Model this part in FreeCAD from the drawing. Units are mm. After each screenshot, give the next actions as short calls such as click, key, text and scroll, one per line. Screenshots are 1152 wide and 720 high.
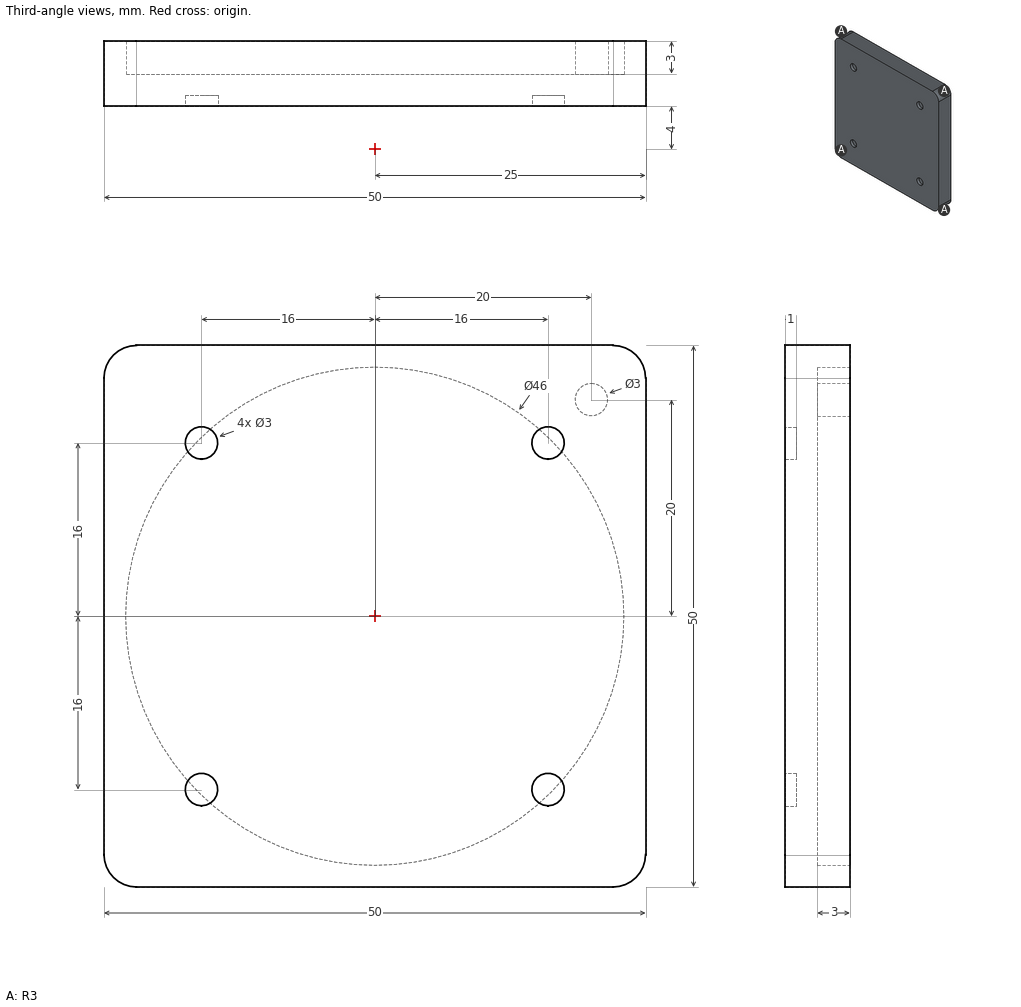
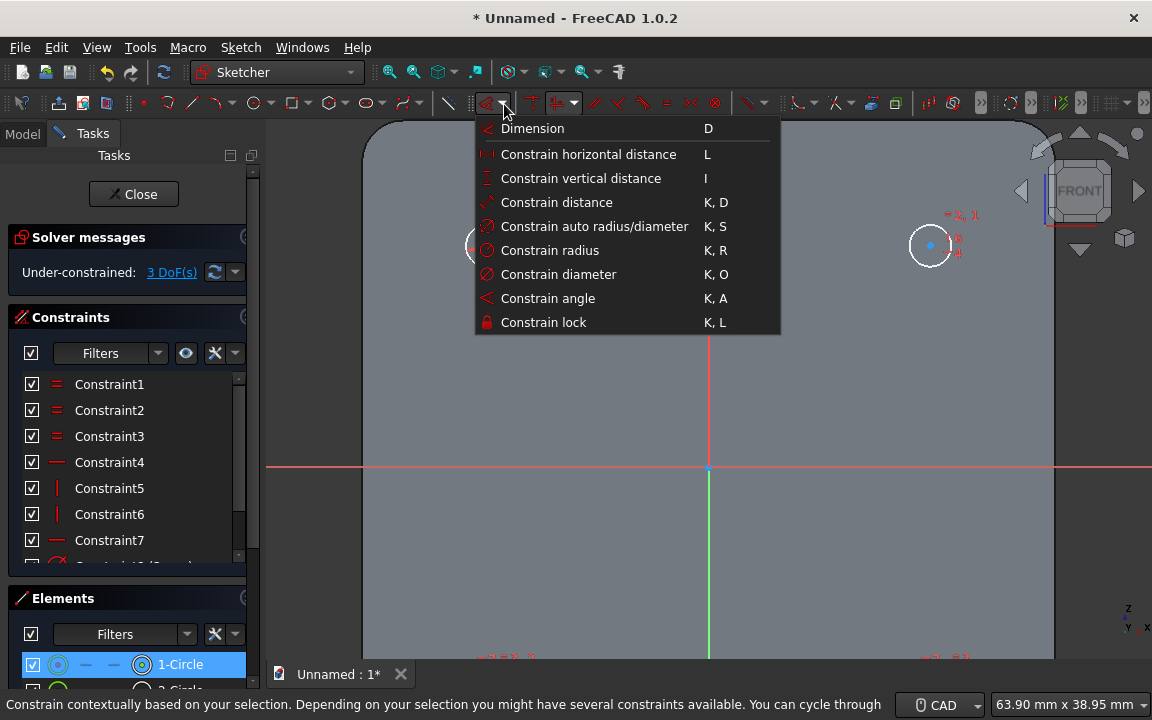
click(628, 178)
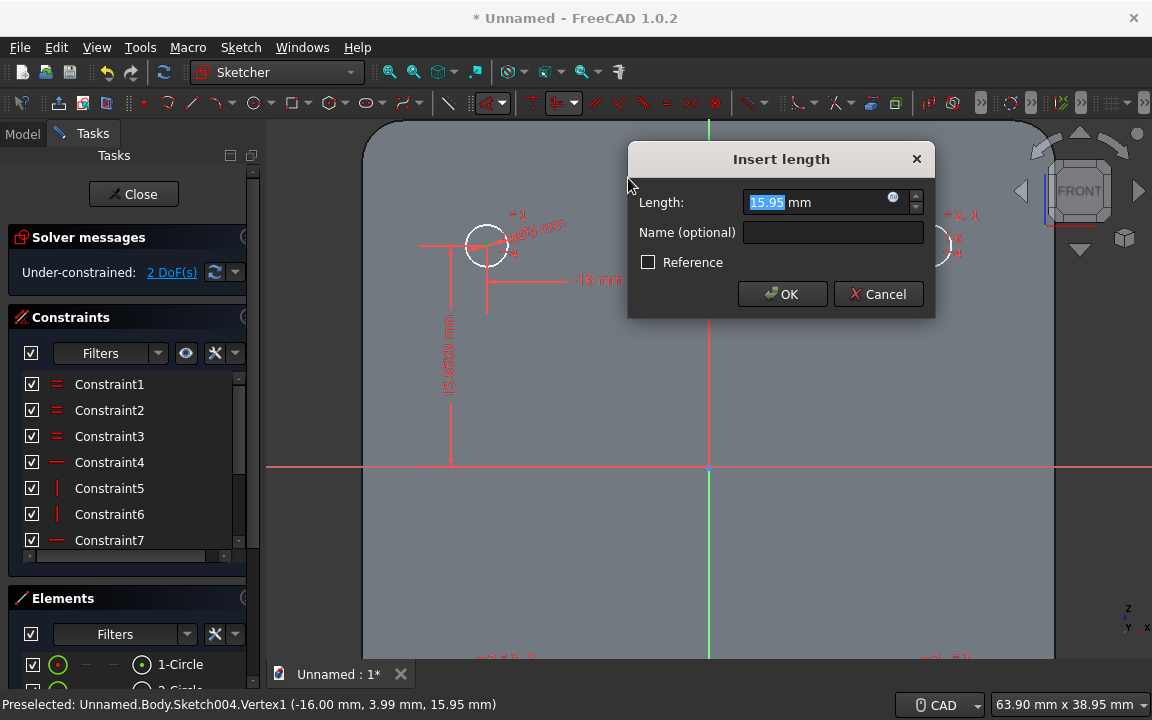
text(16)
key(Return)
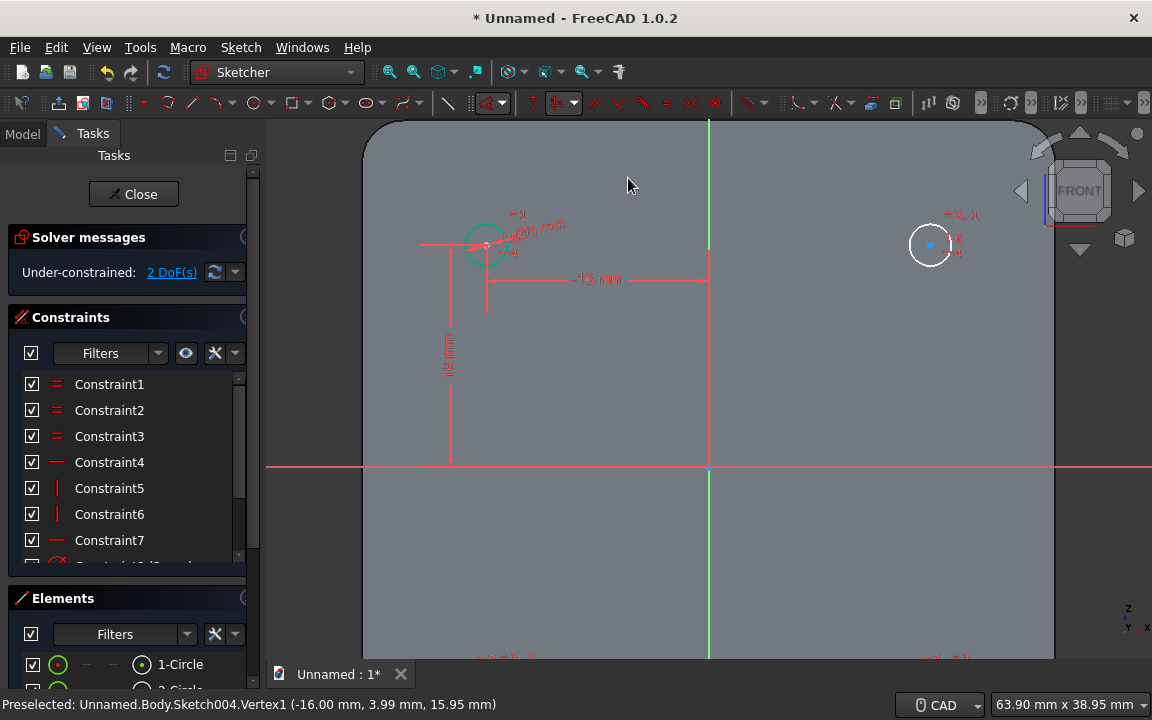
click(930, 245)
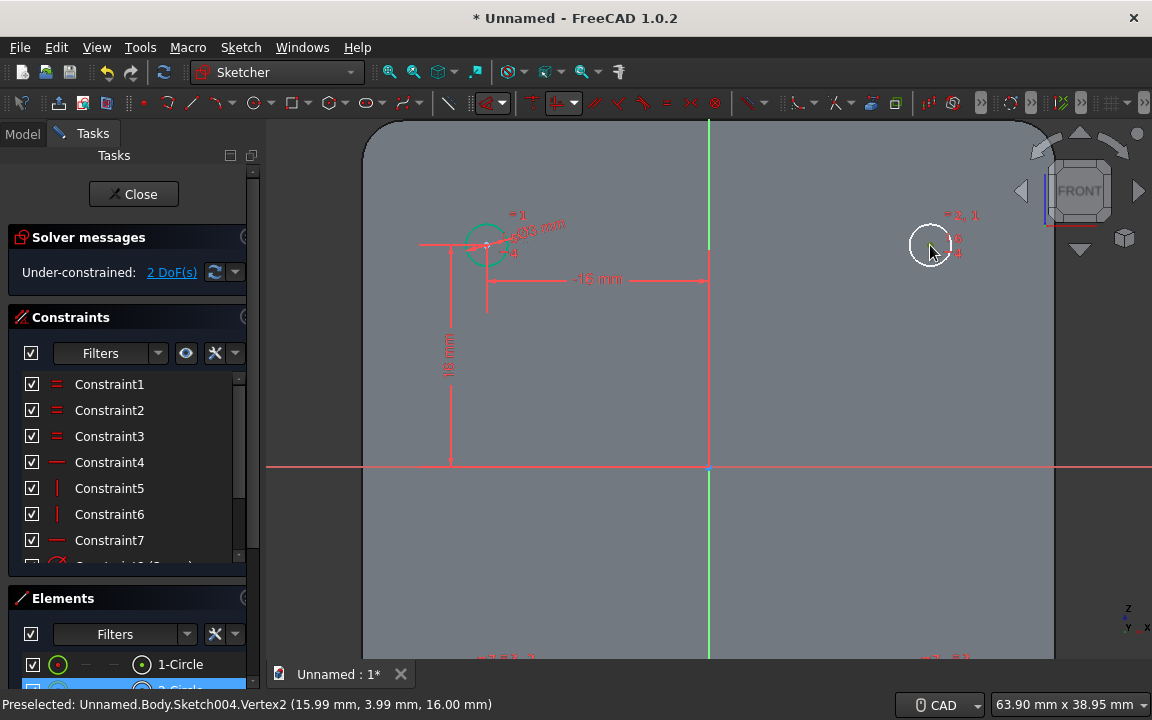
key(l)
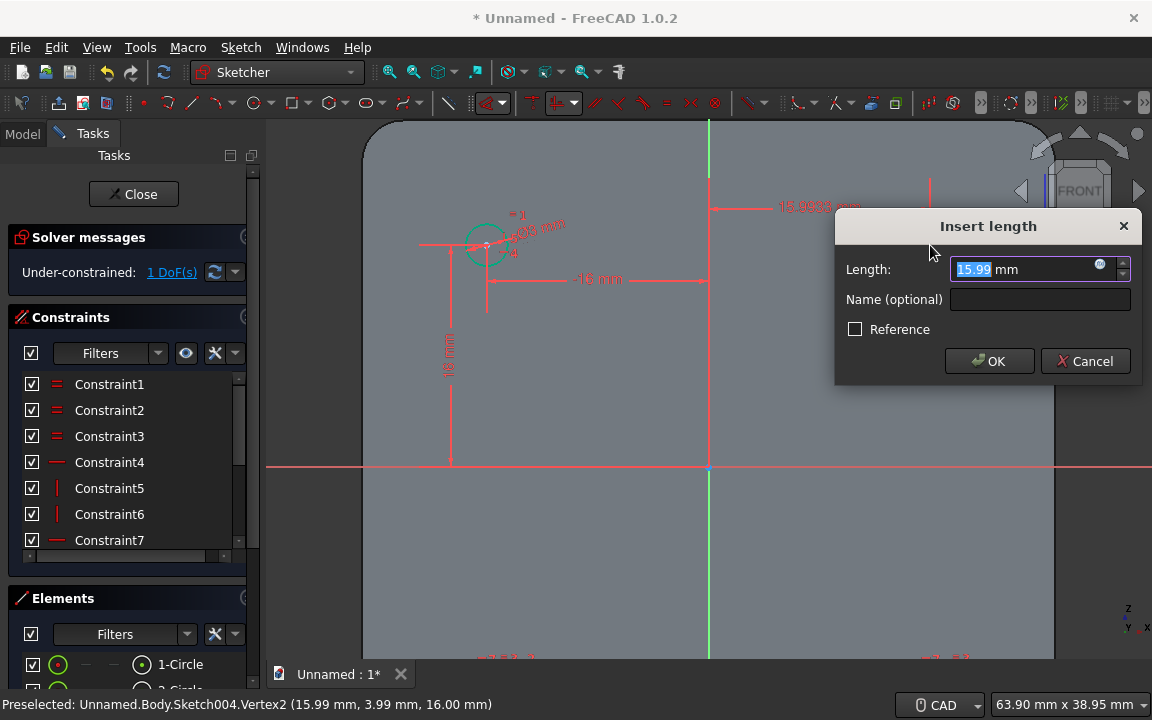
text(16)
key(Return)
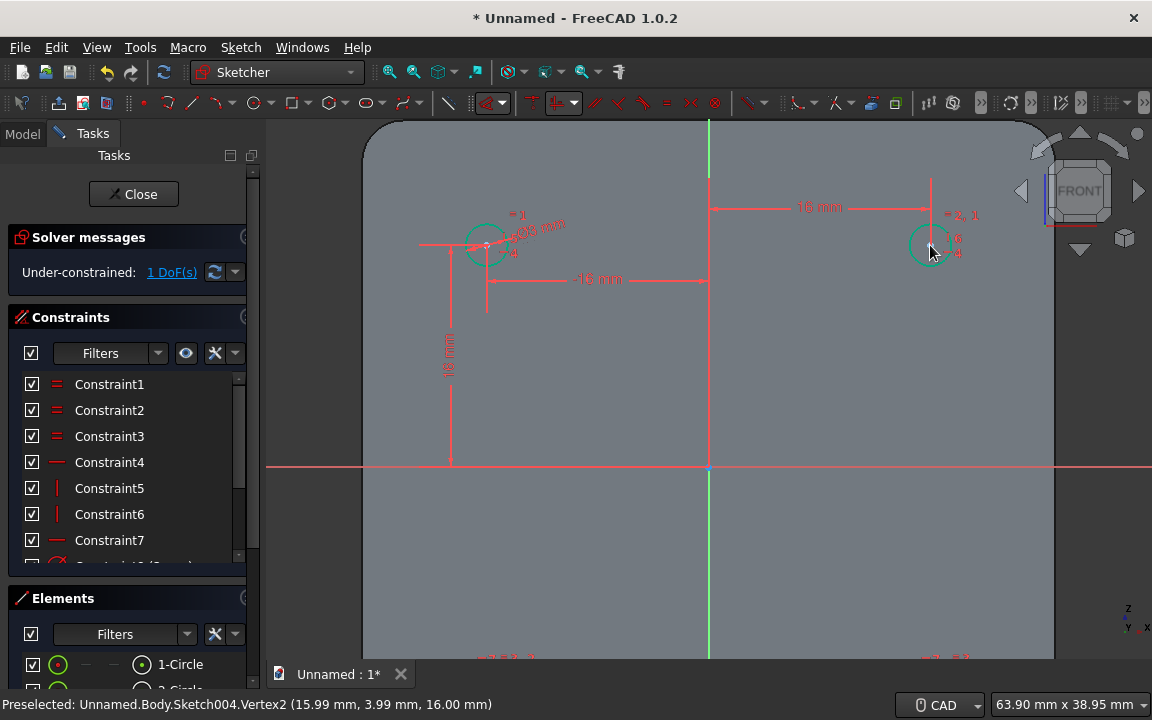
scroll(502, 230, down, 2)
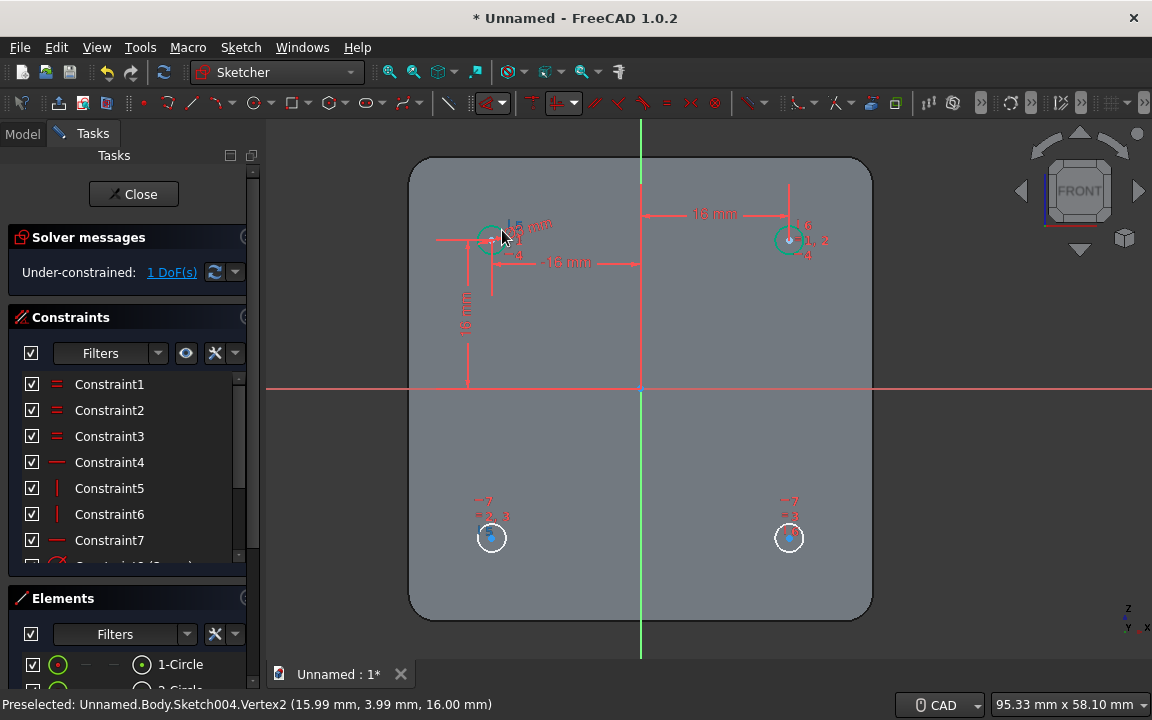
click(492, 538)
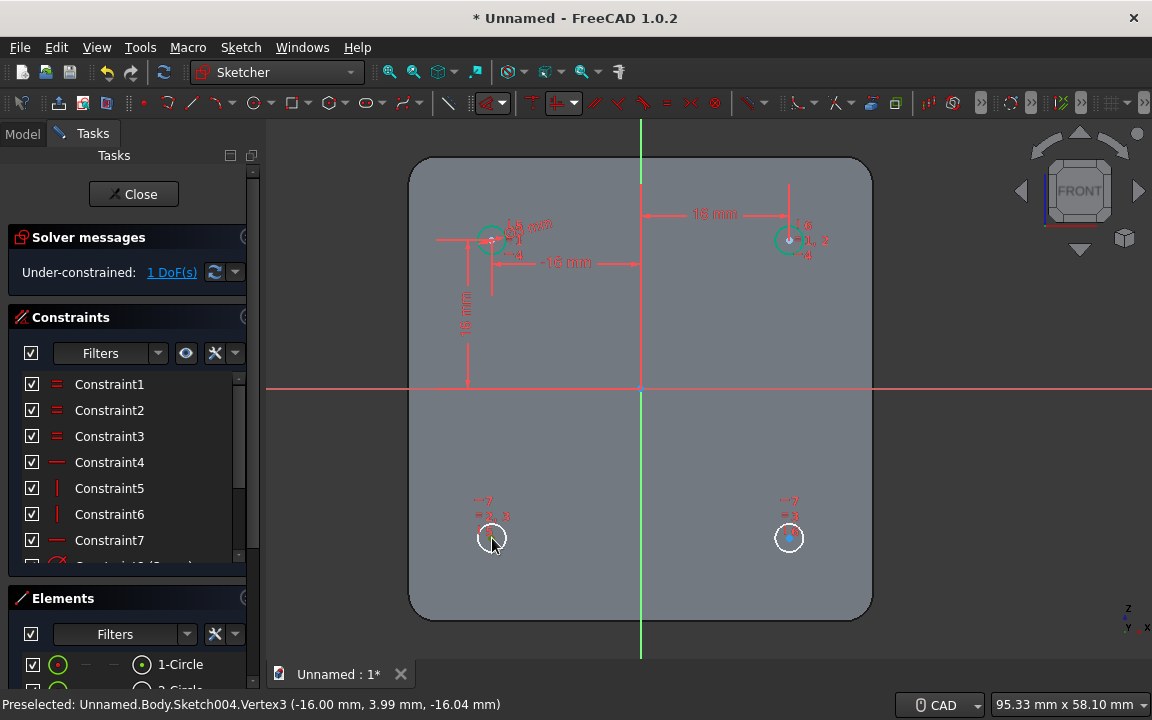
key(i)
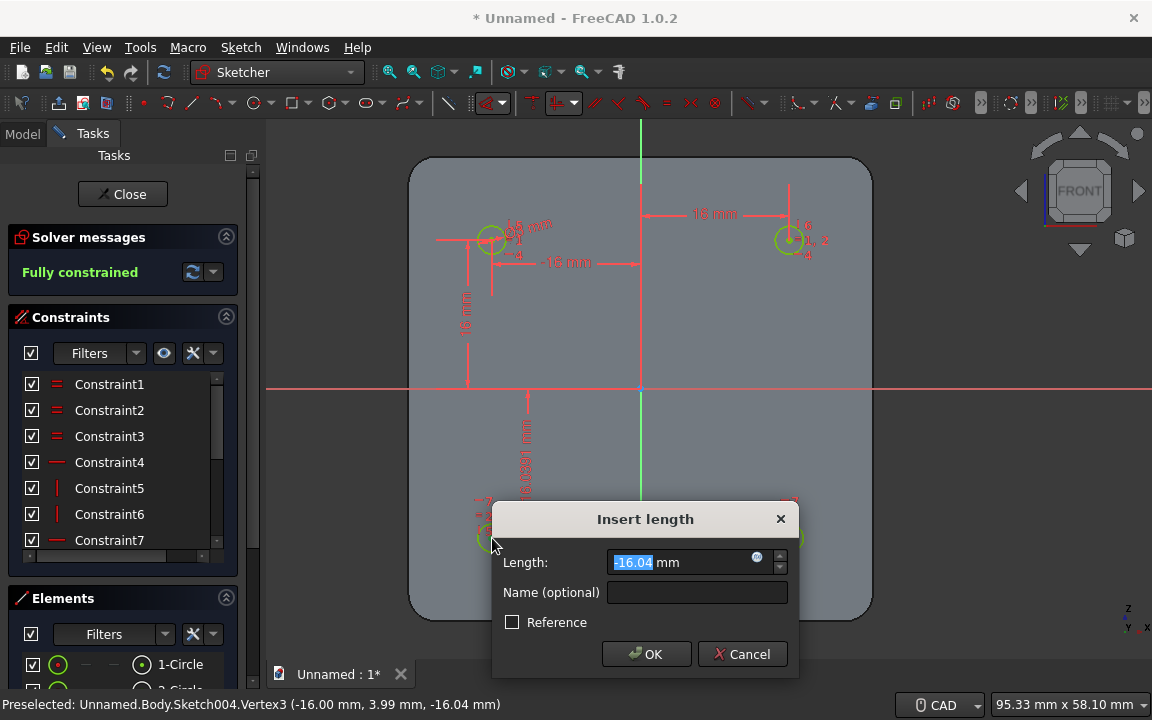
text(-16)
key(Return)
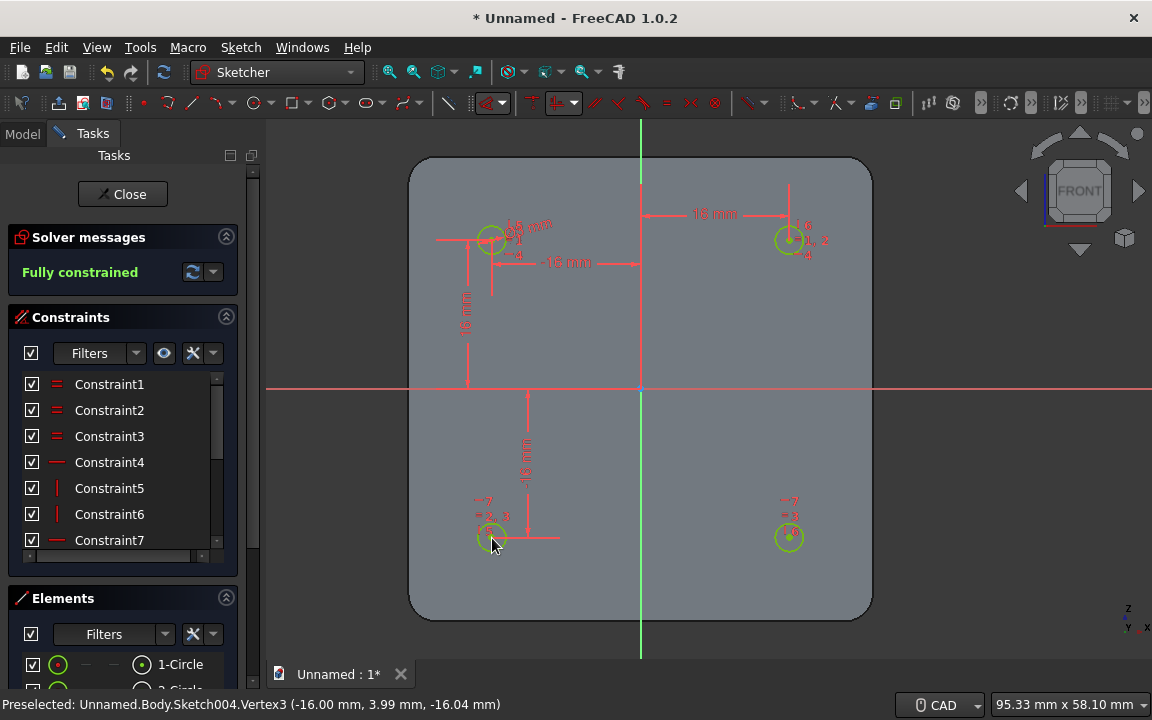
click(123, 194)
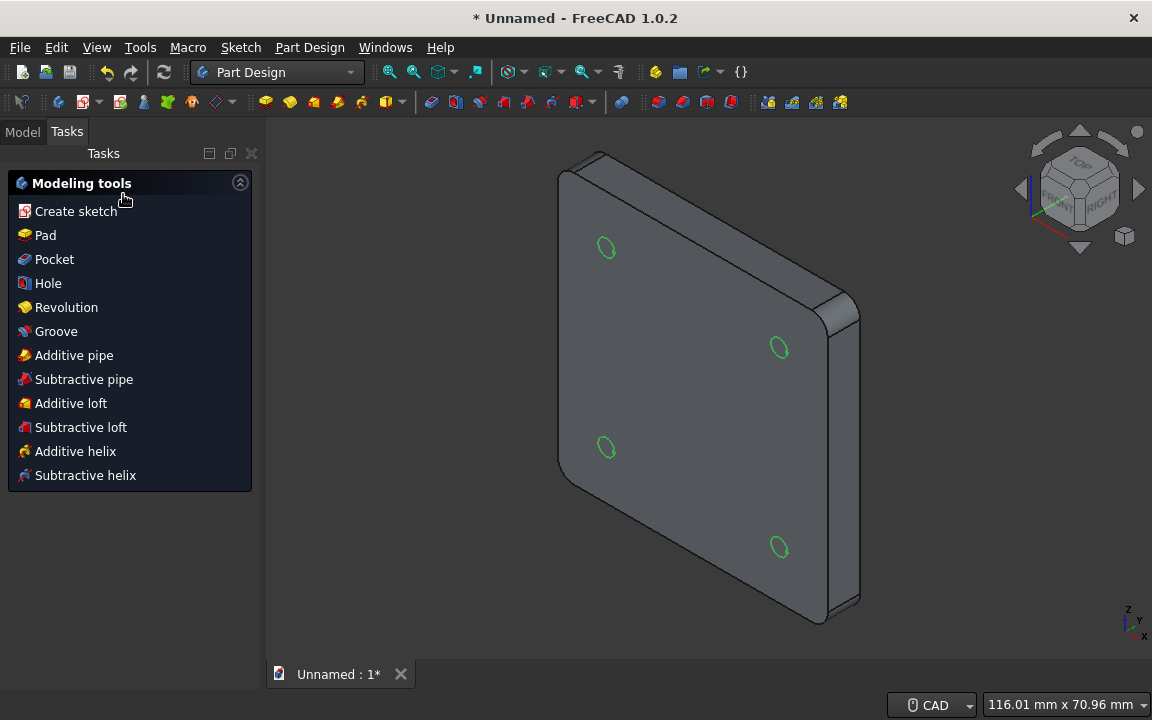
click(432, 102)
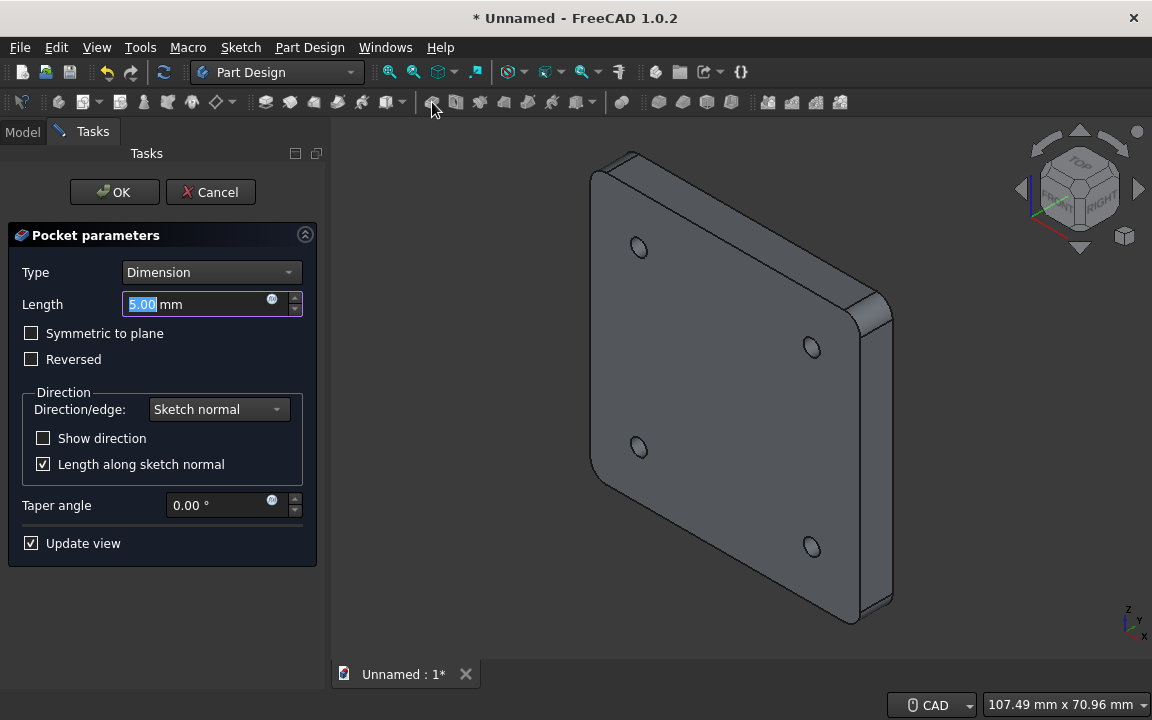
text(1)
key(Tab)